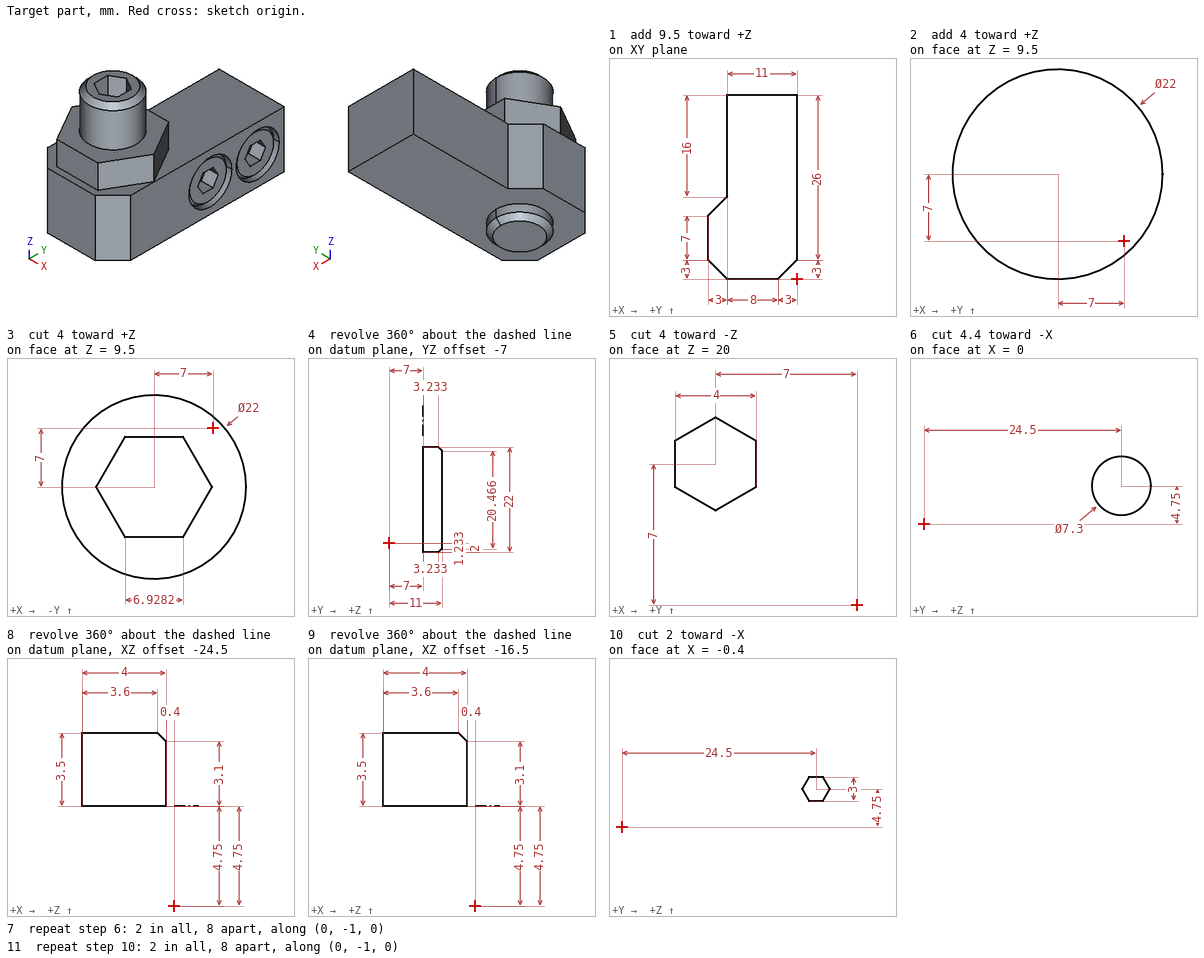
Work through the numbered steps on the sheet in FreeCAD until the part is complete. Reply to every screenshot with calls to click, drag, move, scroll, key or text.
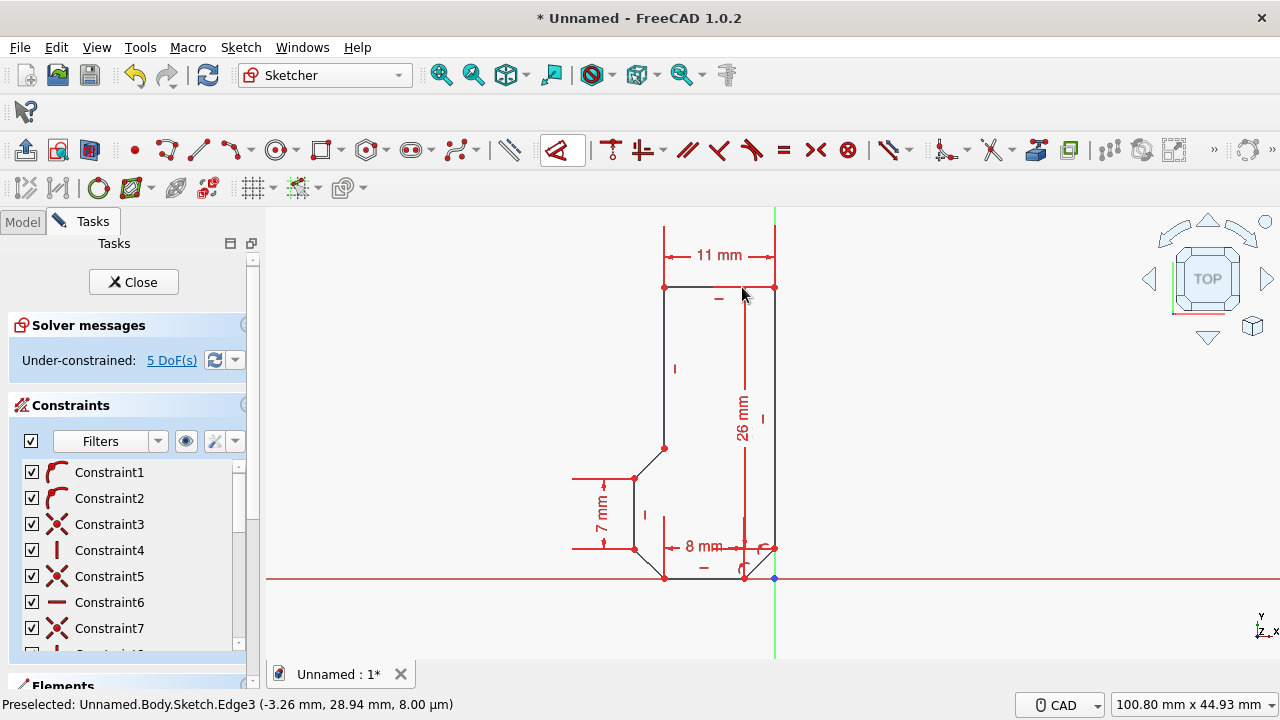
click(664, 336)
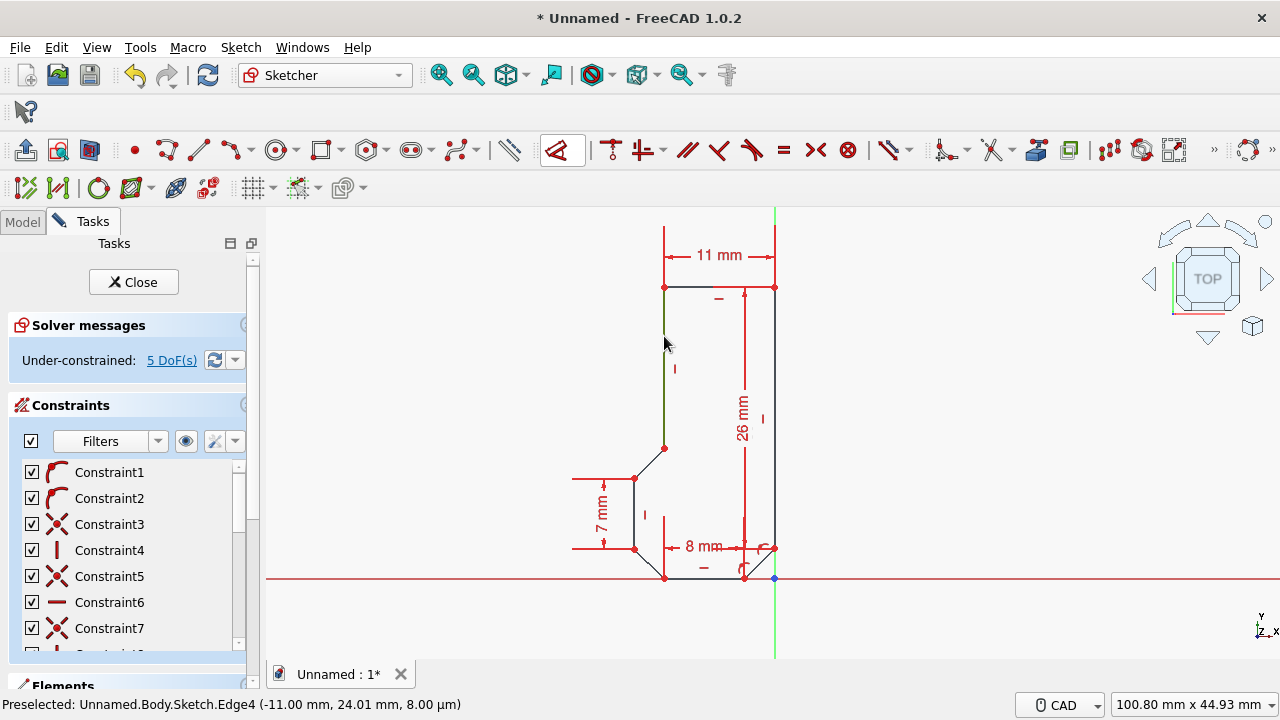
click(580, 150)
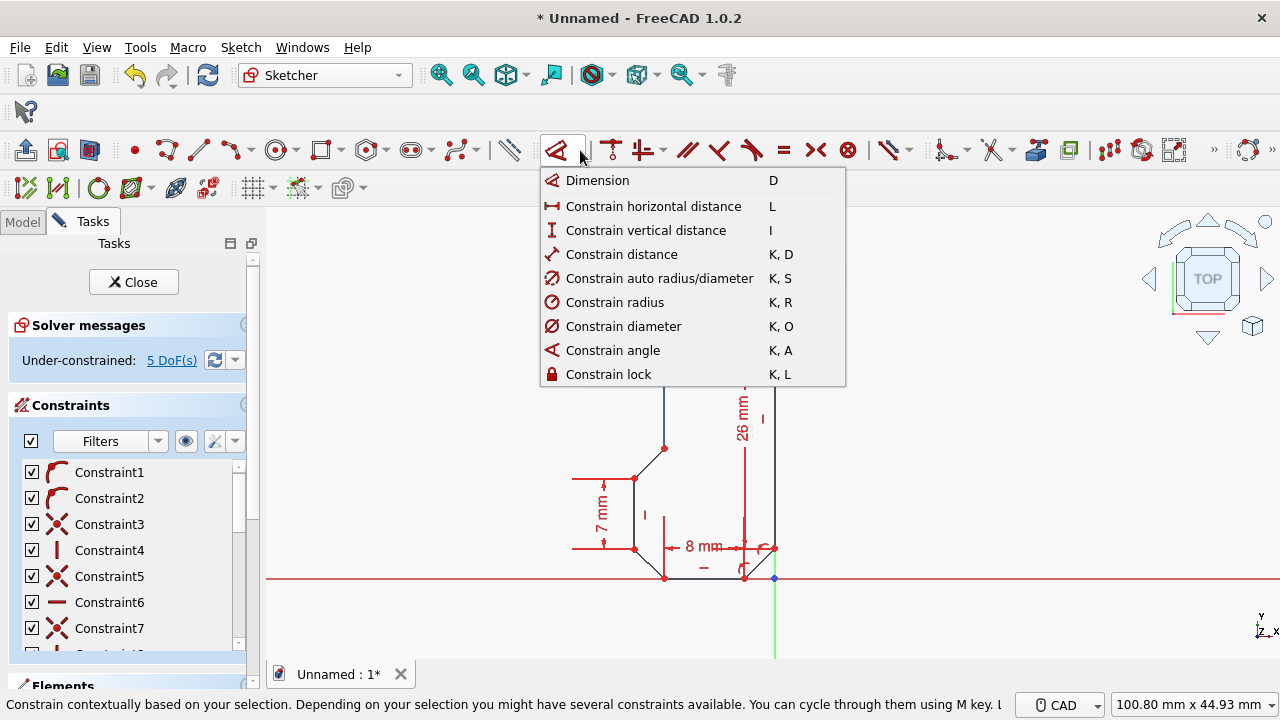
click(693, 230)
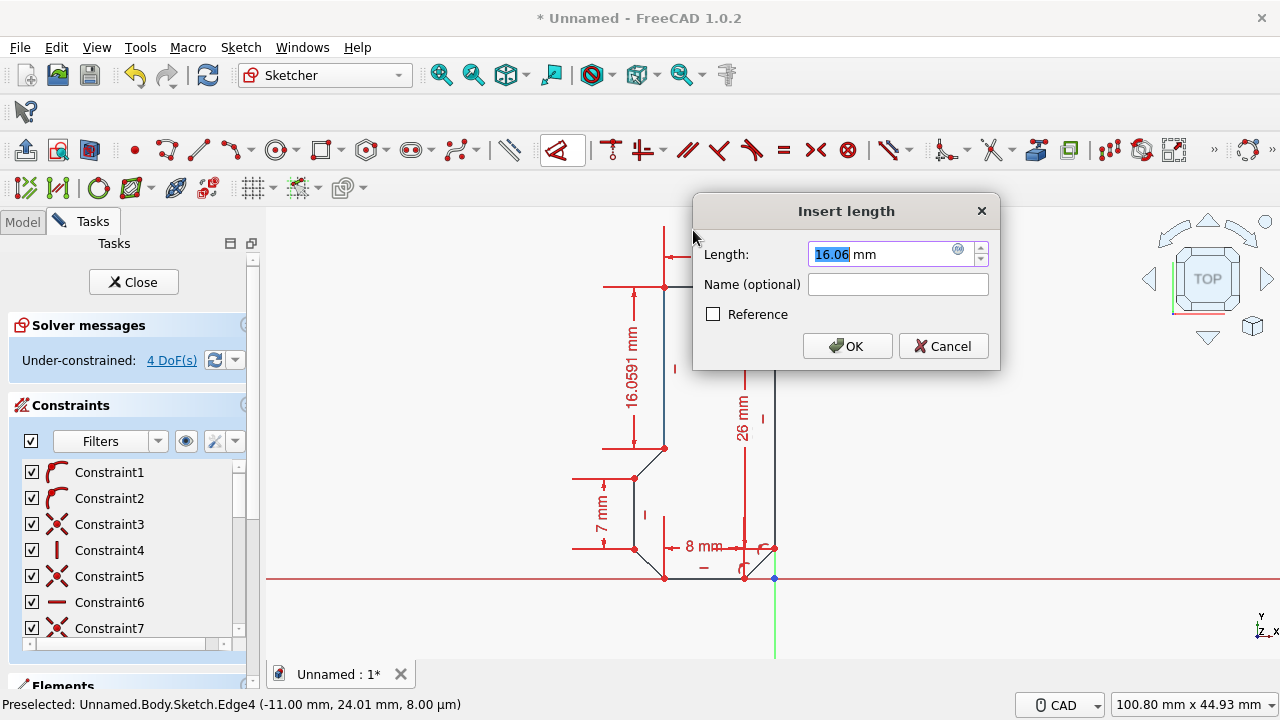
text(16)
key(Return)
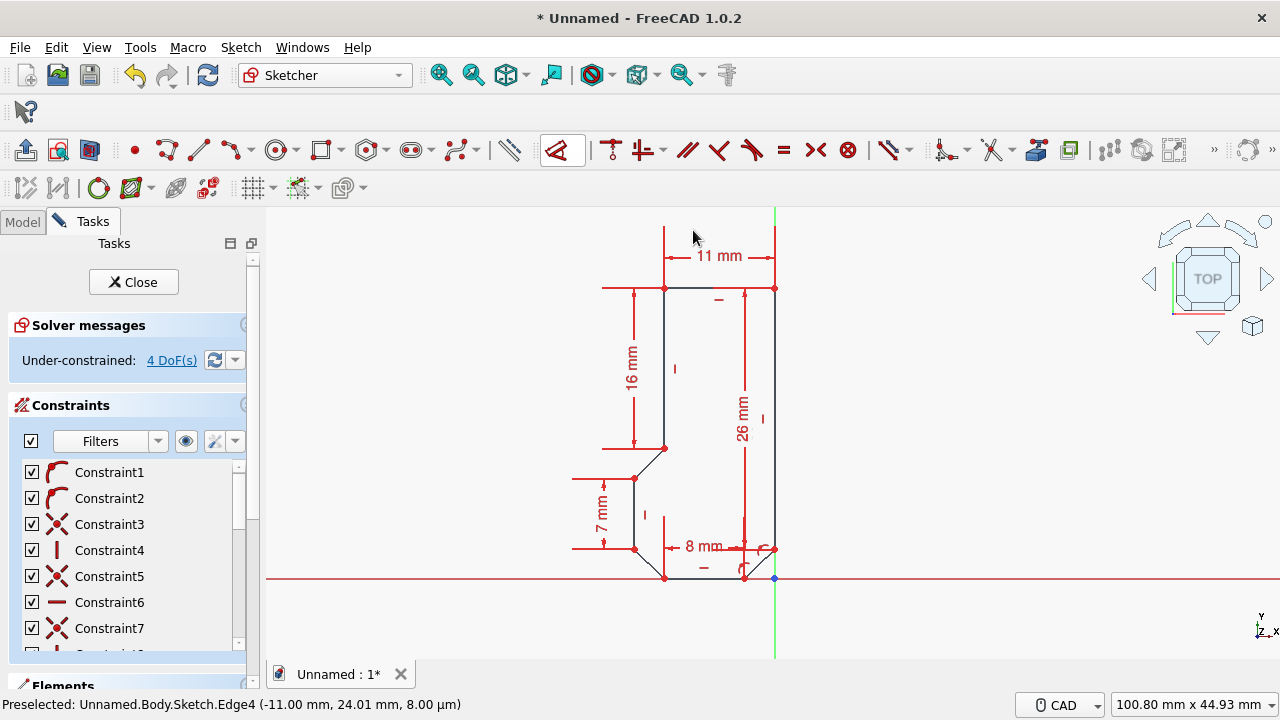
scroll(744, 579, up, 2)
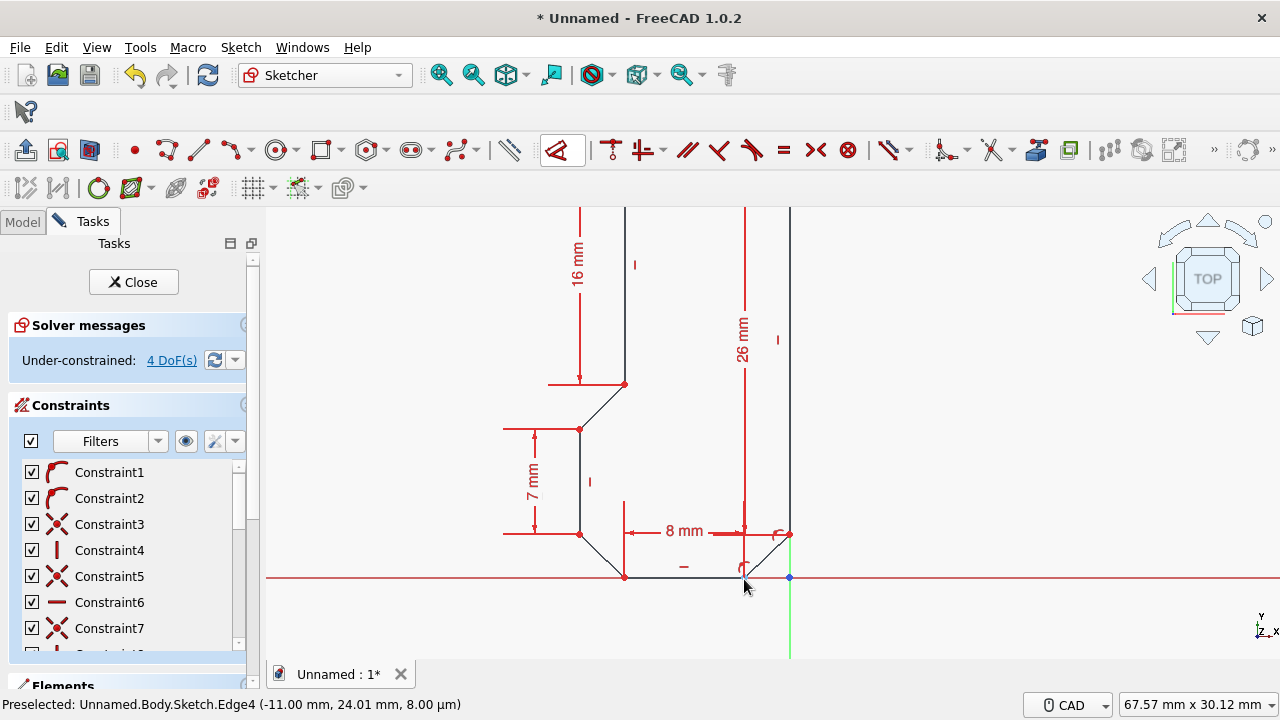
click(744, 578)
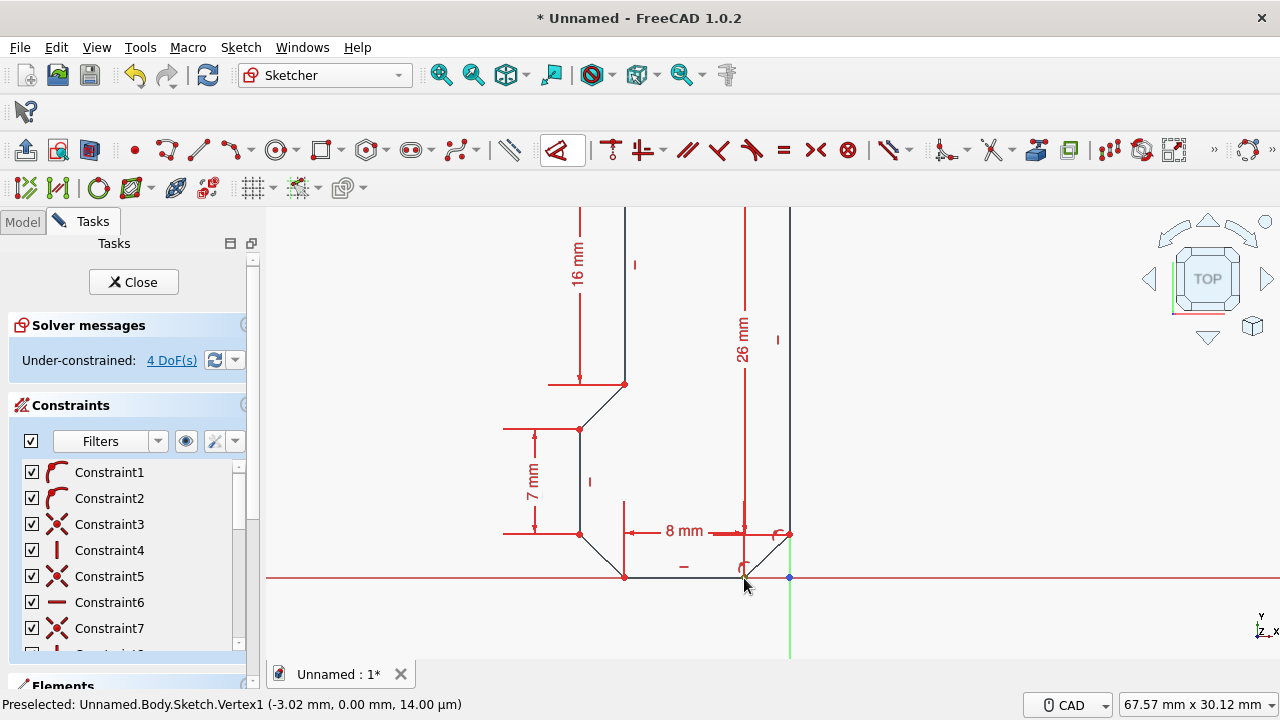
key(l)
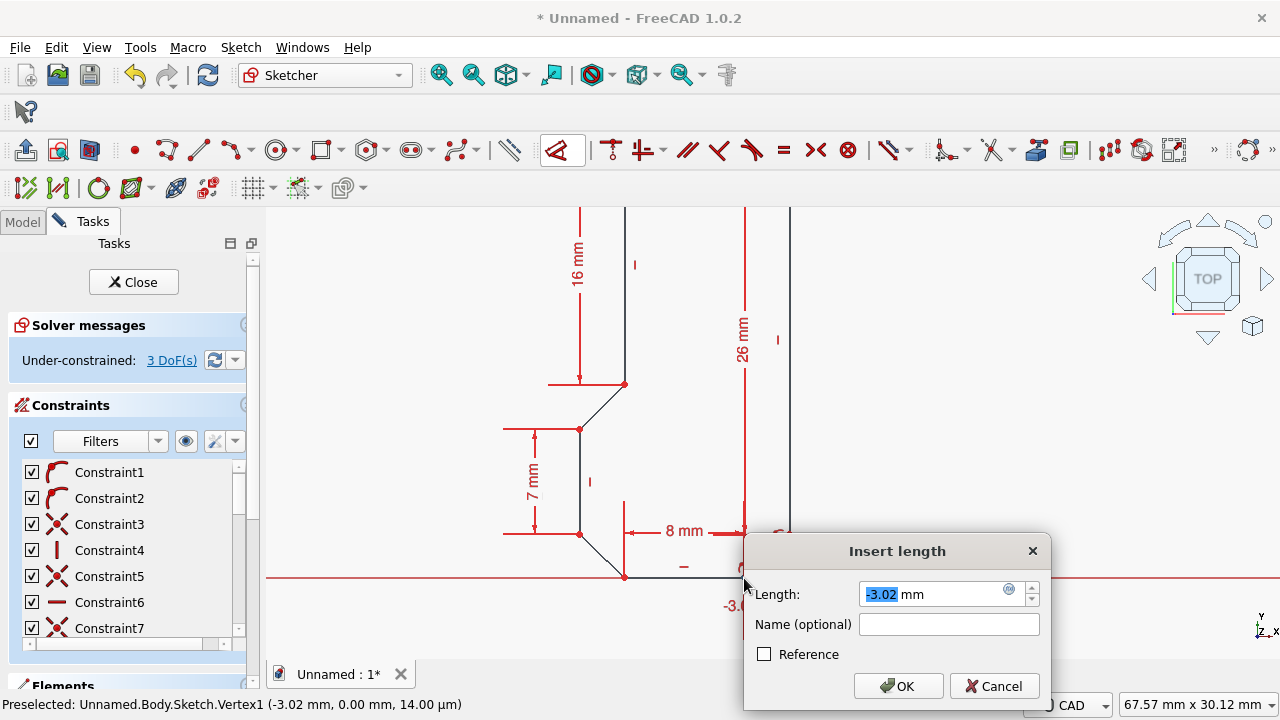
text(-3)
key(Return)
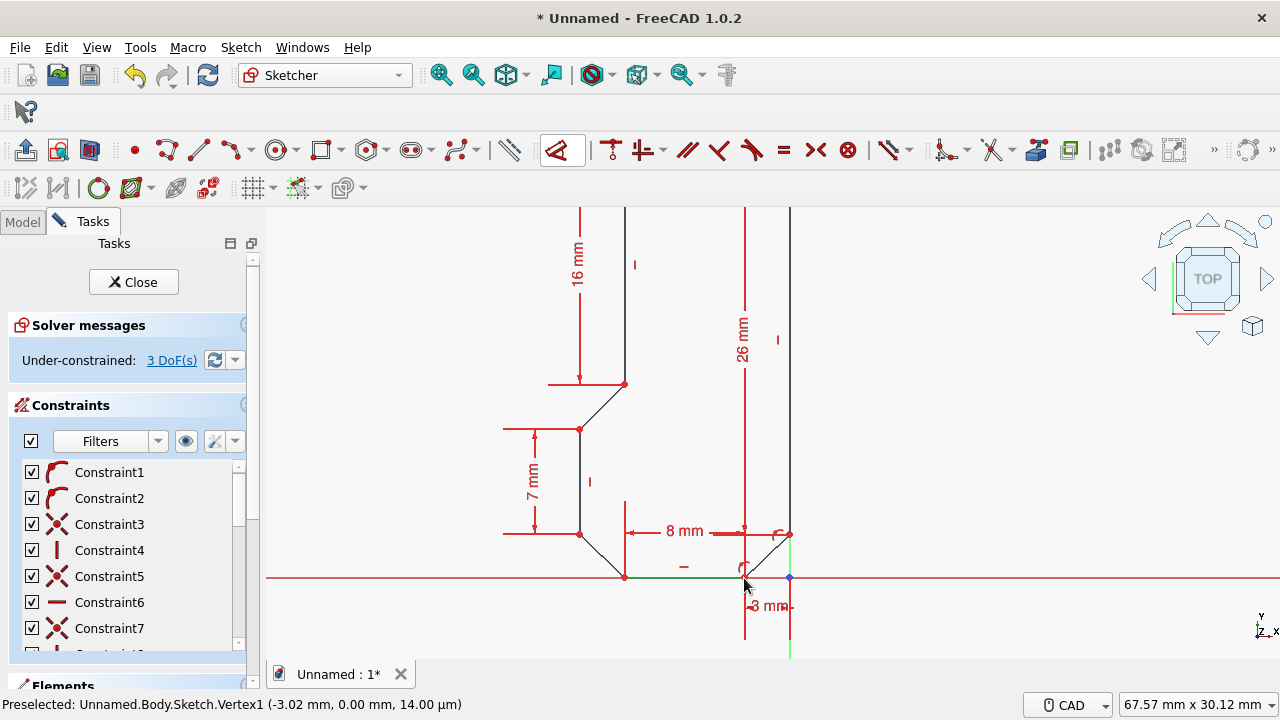
click(790, 535)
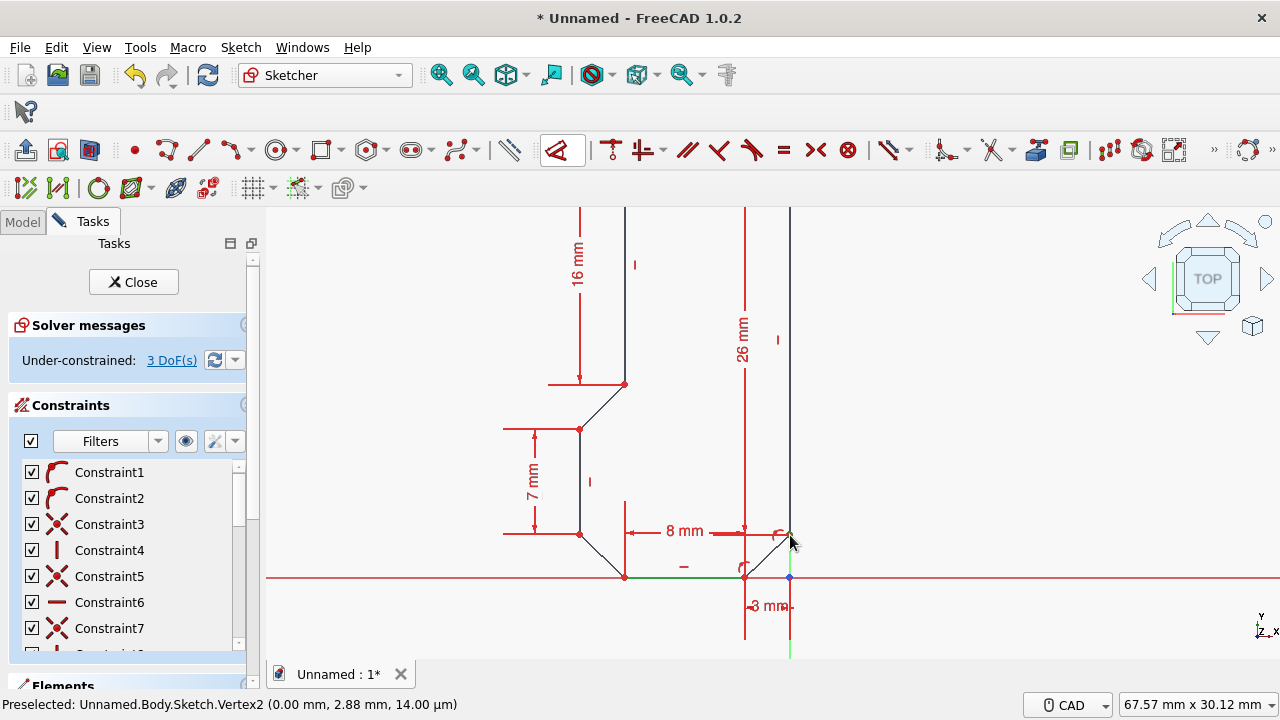
key(i)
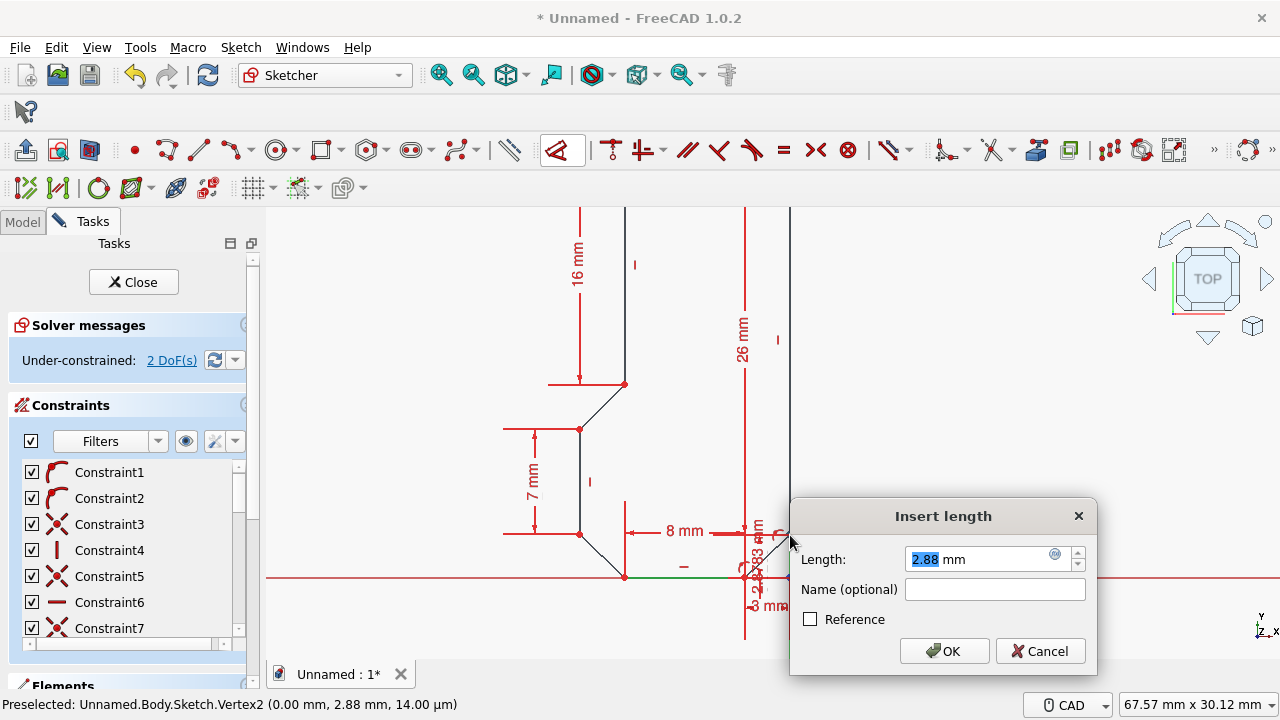
text(3)
key(Return)